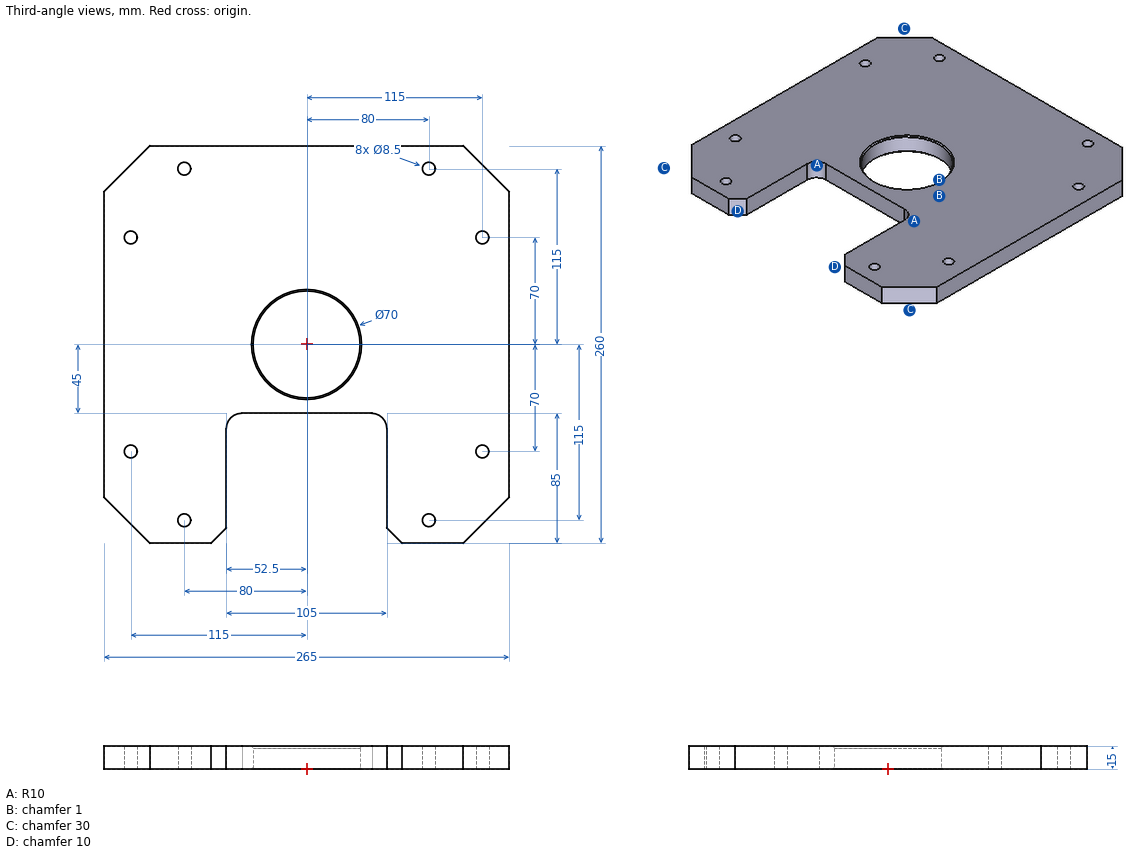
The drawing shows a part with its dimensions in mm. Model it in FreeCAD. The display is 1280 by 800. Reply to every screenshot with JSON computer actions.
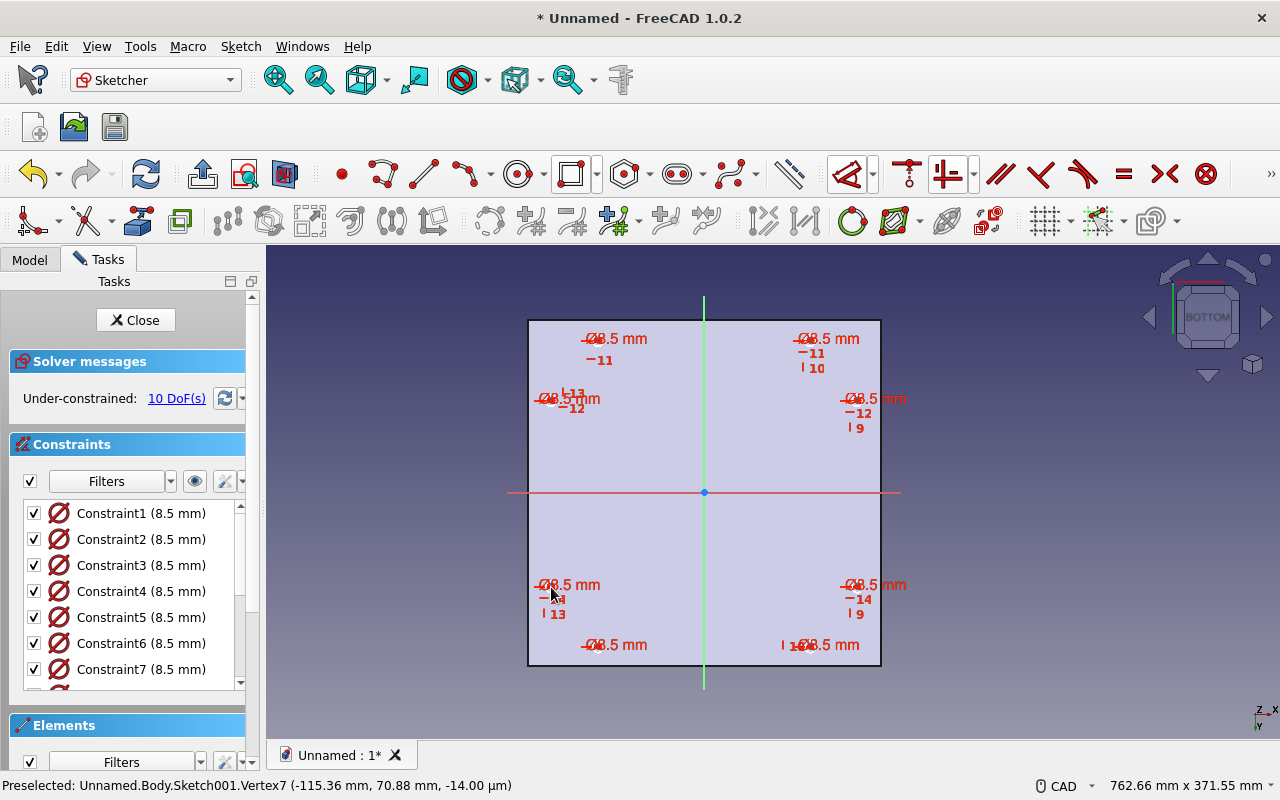
{"action": "left_click", "coordinate": [598, 341]}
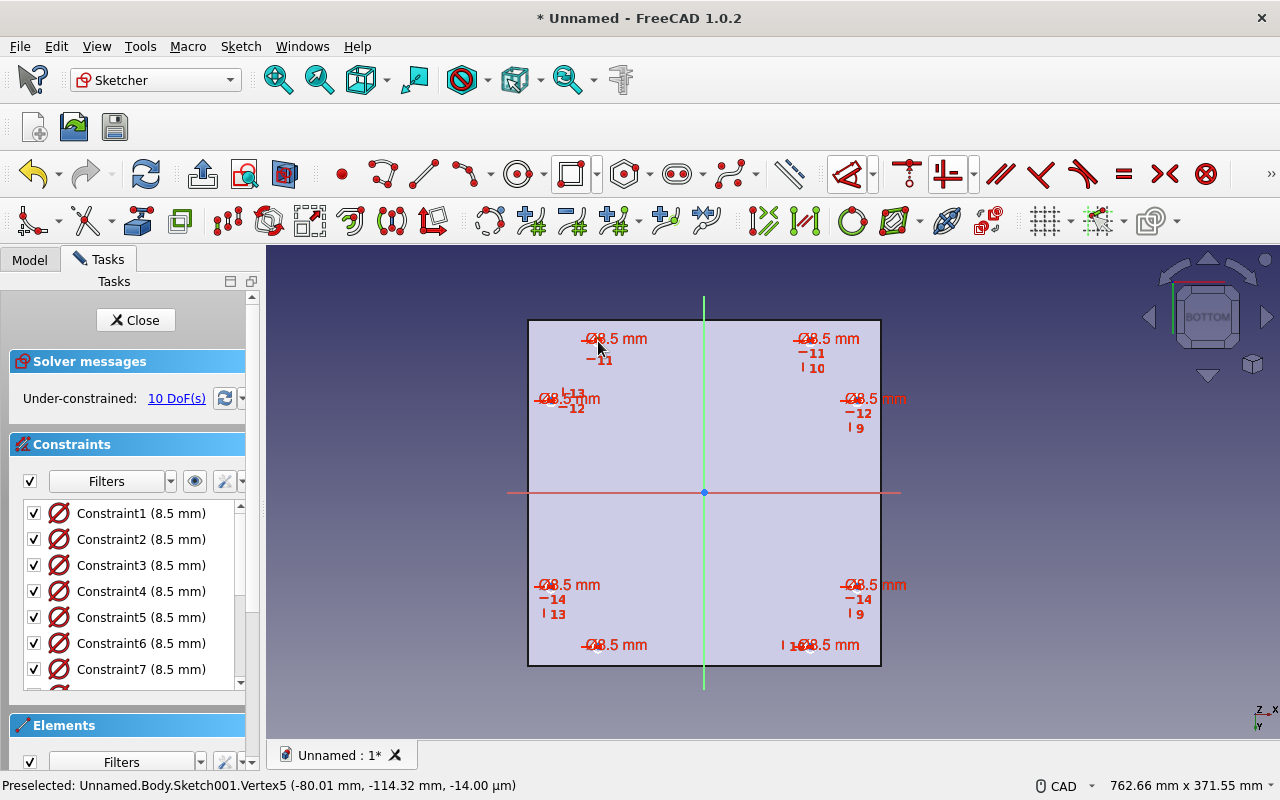
{"action": "left_click", "coordinate": [598, 647]}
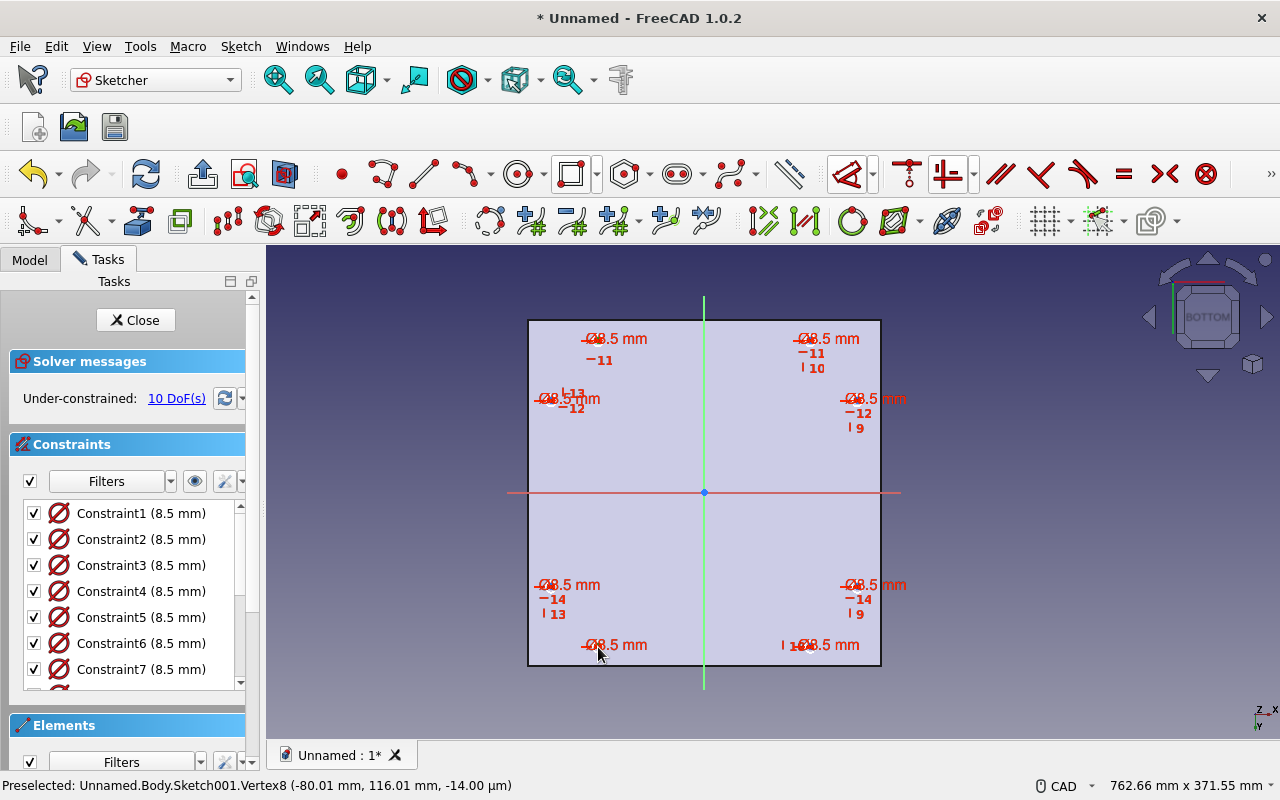
{"action": "key", "text": "v"}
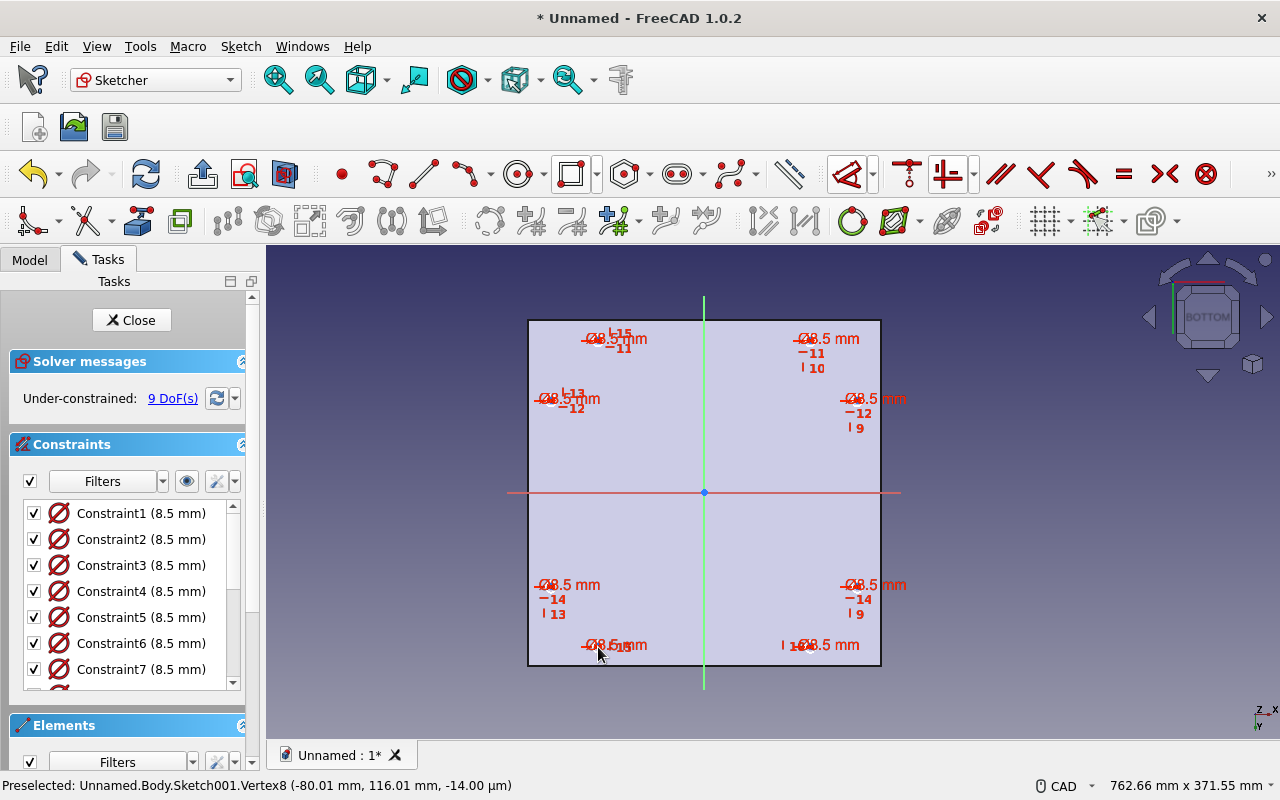
{"action": "left_click", "coordinate": [810, 647]}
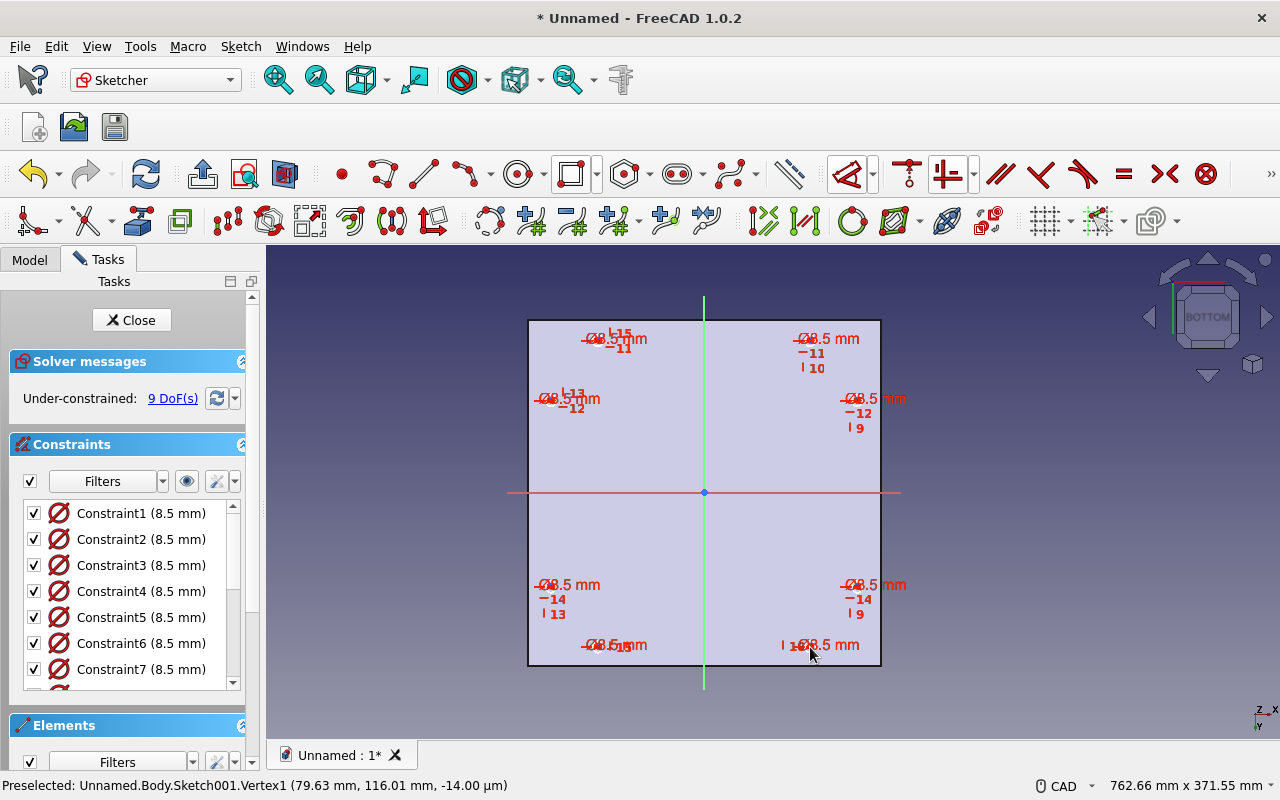
{"action": "left_click", "coordinate": [598, 647]}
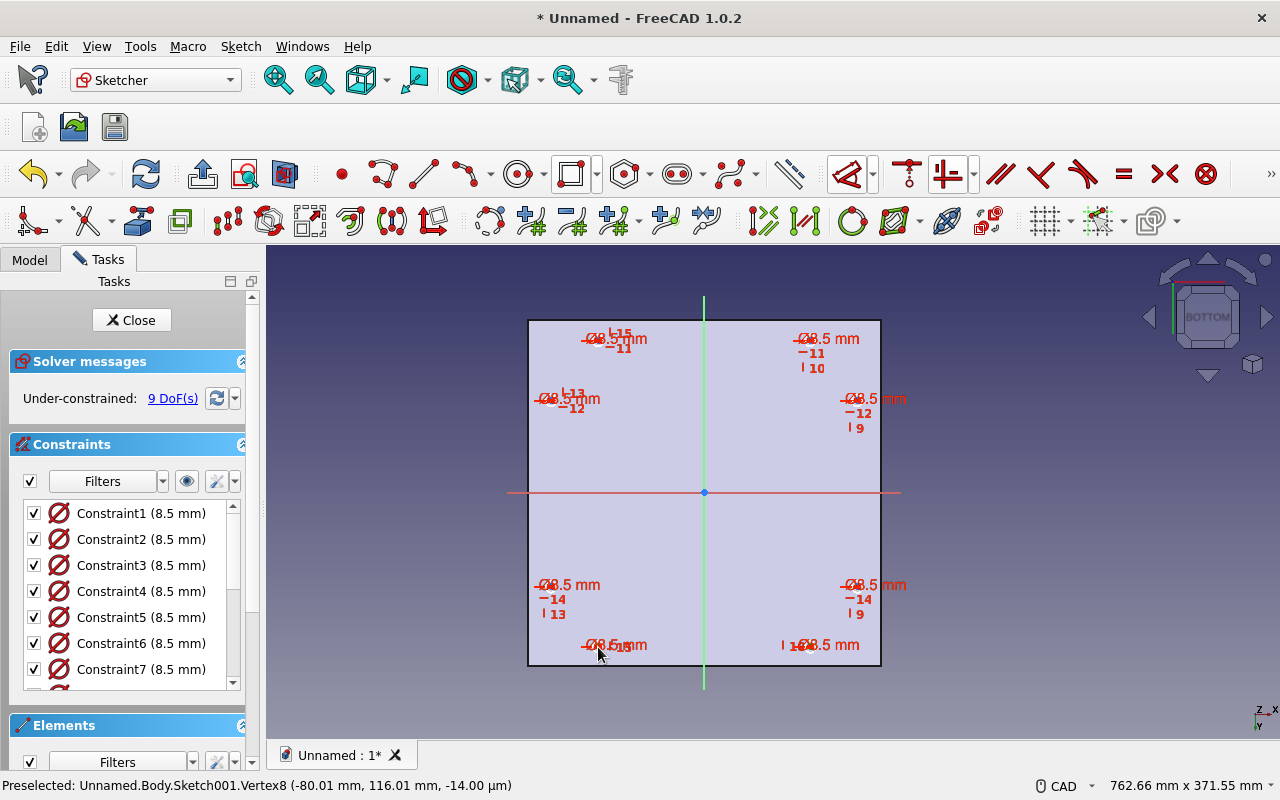
{"action": "key", "text": "h"}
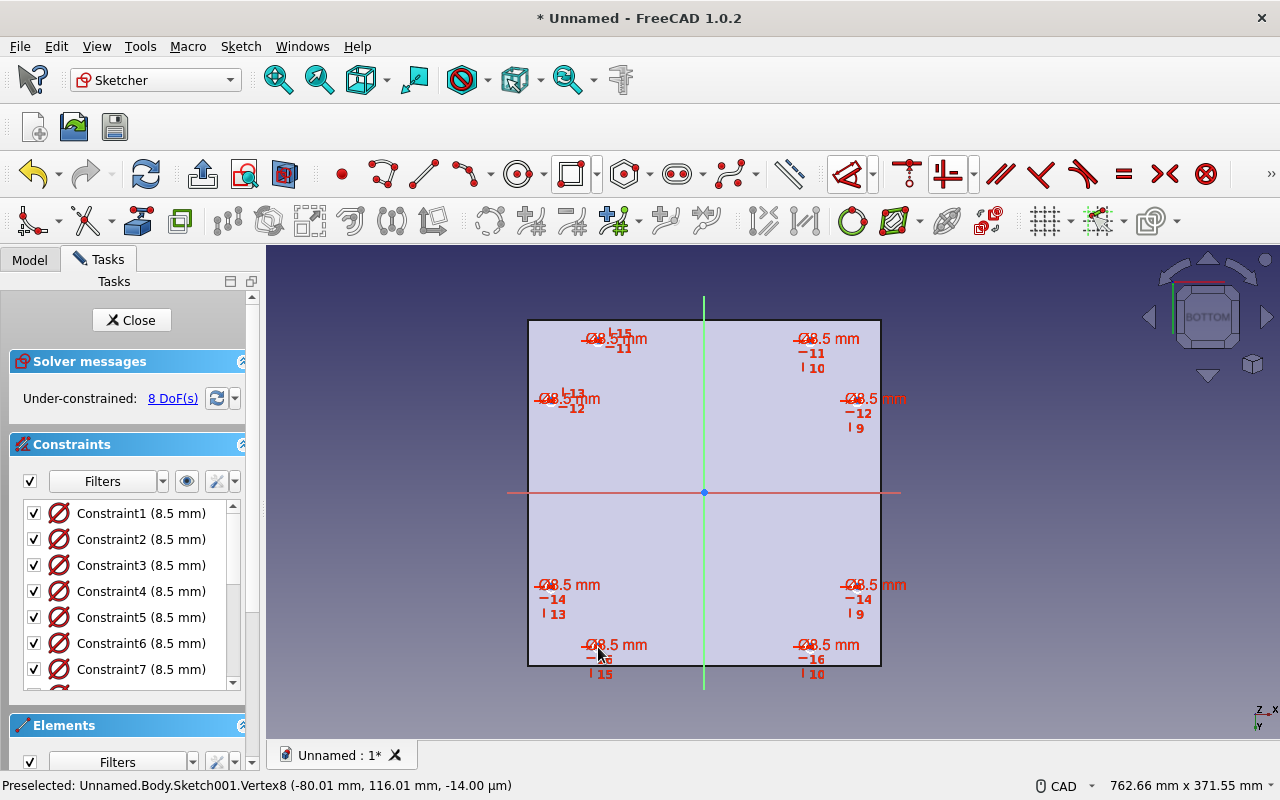
{"action": "left_click", "coordinate": [846, 174]}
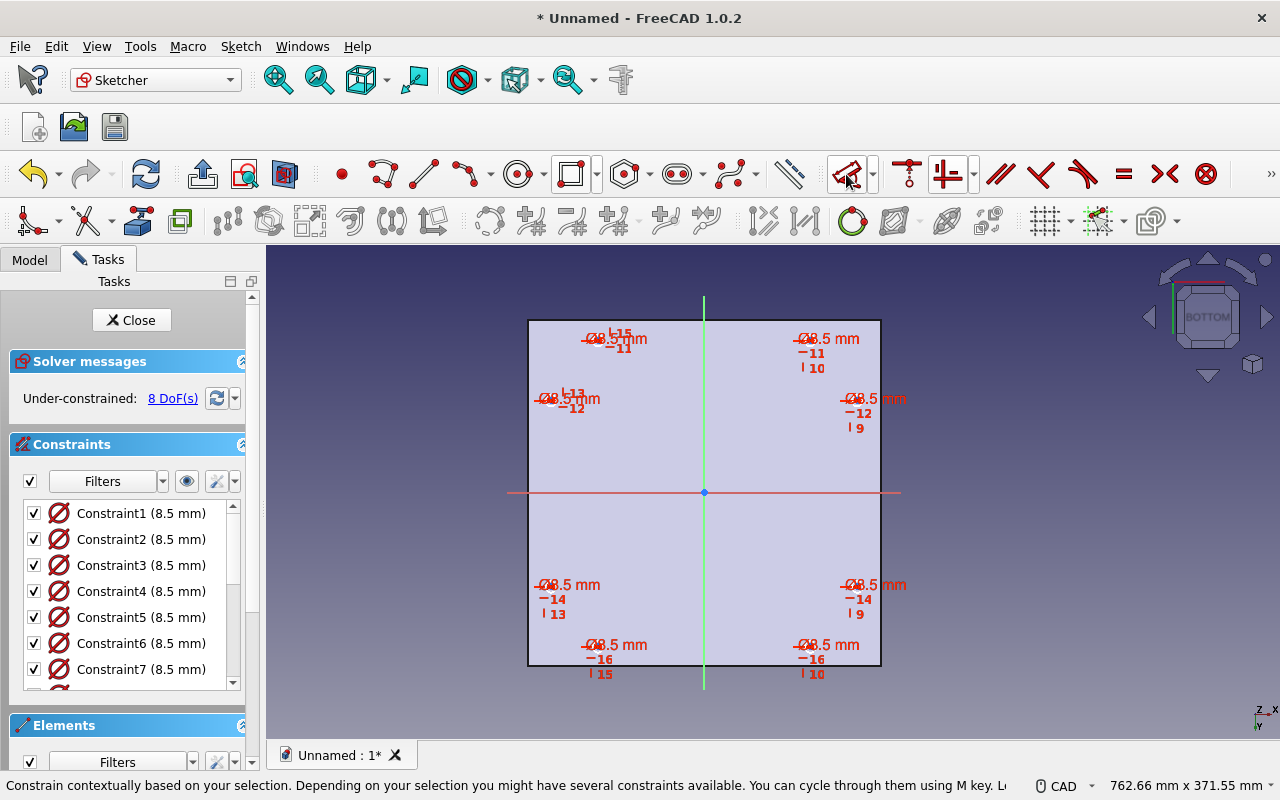
{"action": "left_click", "coordinate": [810, 647]}
{"action": "left_click", "coordinate": [757, 681]}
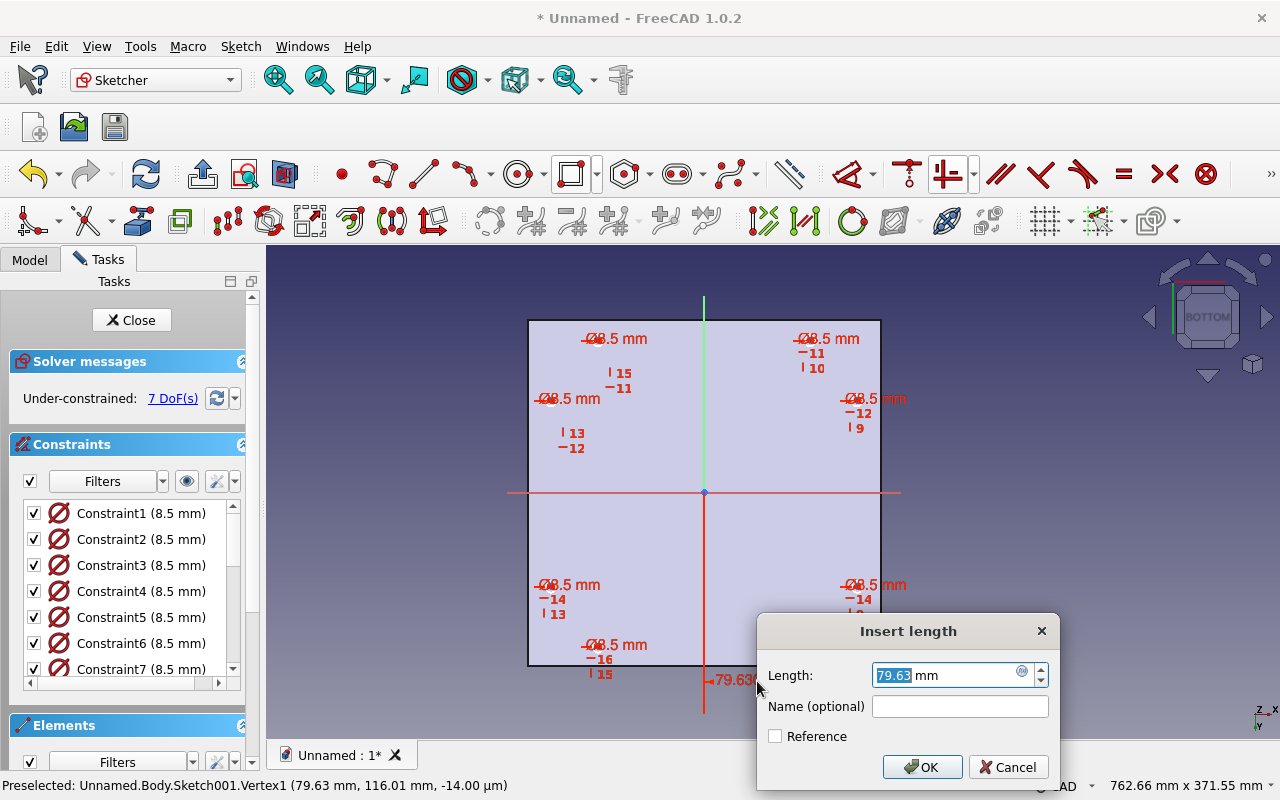
{"action": "type", "text": "80"}
{"action": "key", "text": "Return"}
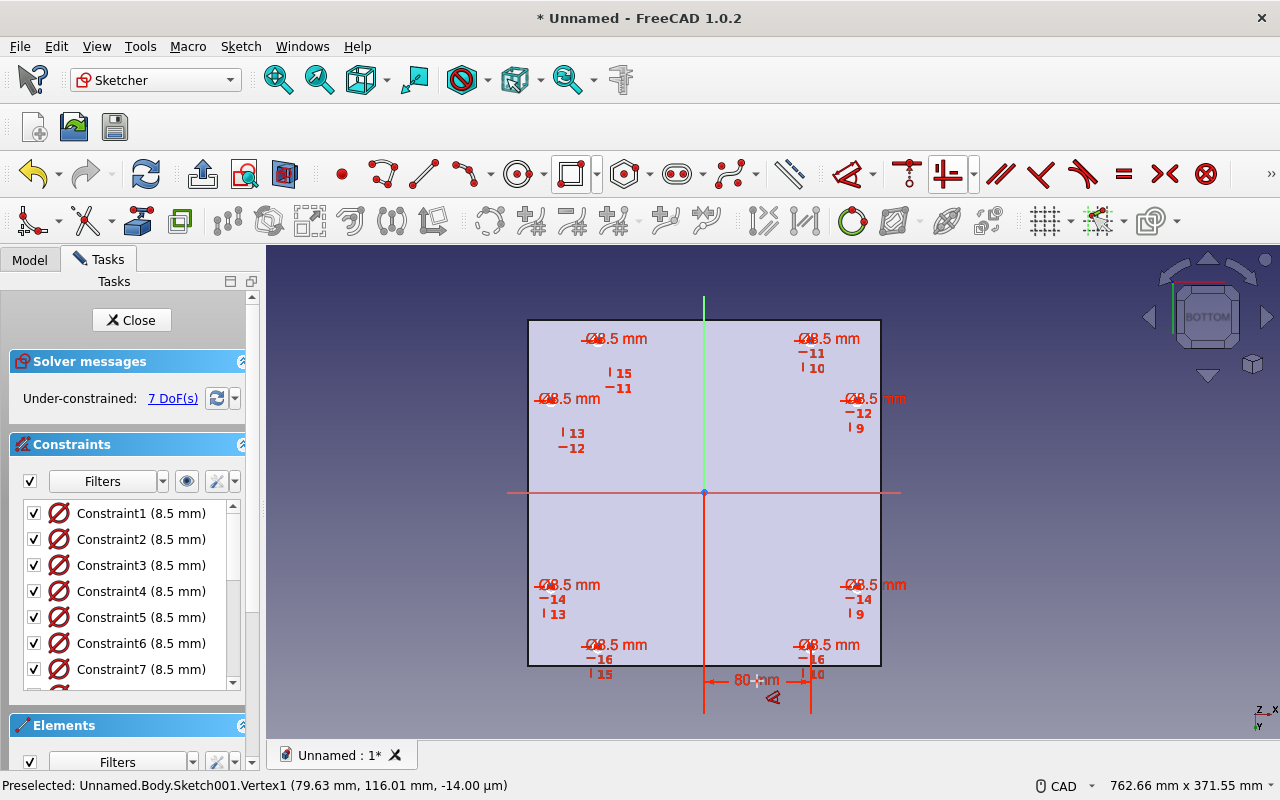
{"action": "left_click", "coordinate": [857, 587]}
{"action": "left_click", "coordinate": [891, 540]}